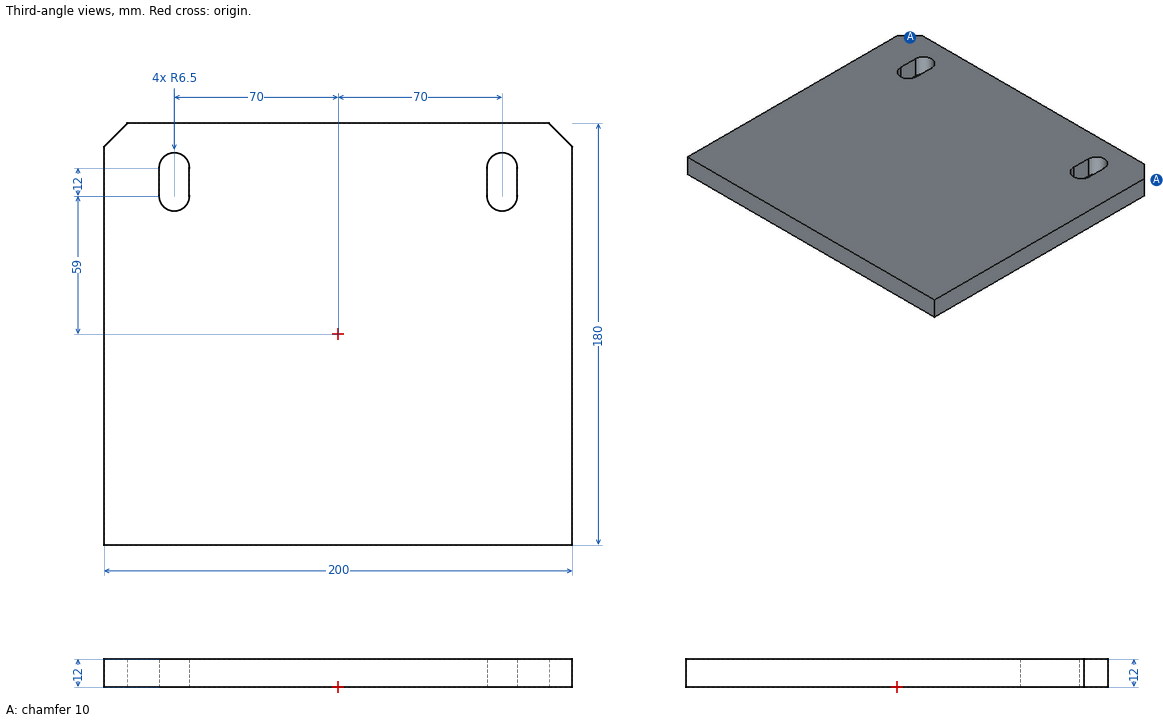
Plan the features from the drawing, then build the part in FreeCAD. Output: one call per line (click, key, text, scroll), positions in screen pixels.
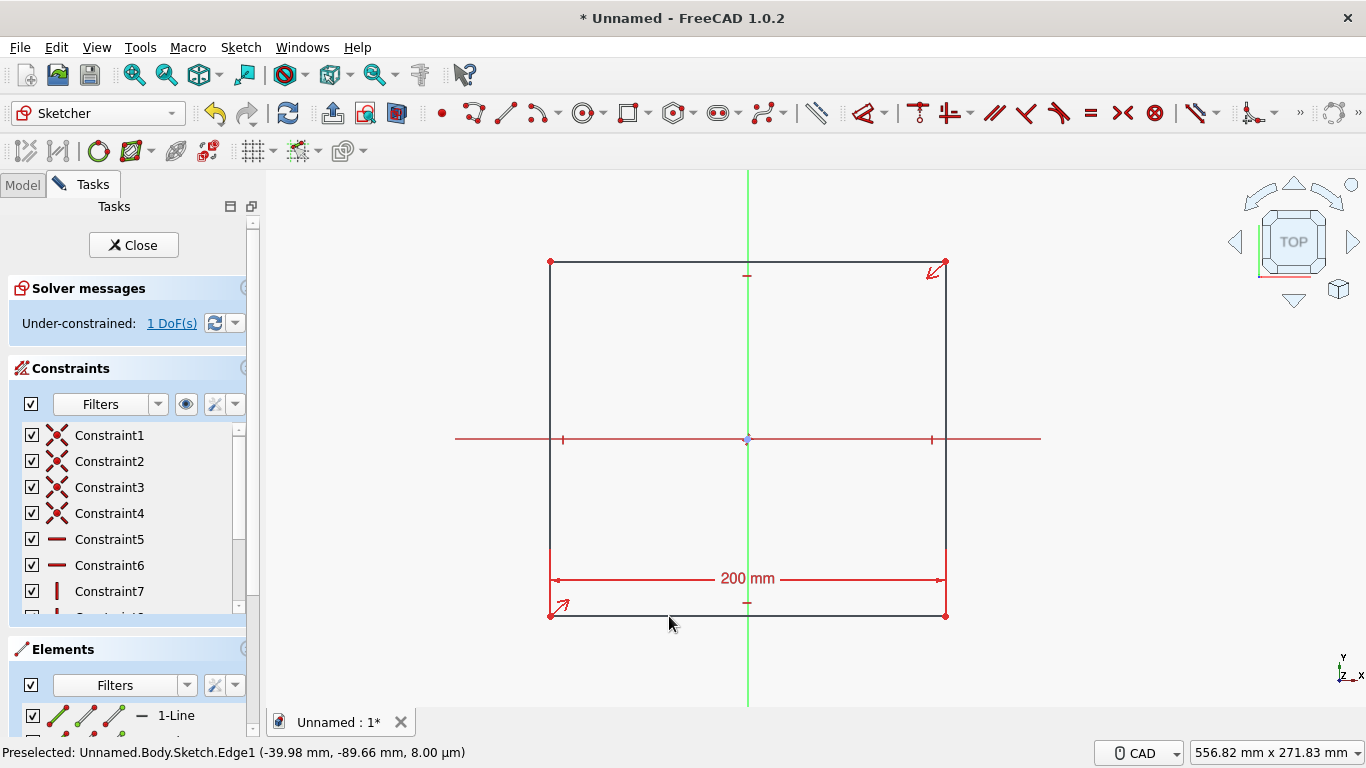
click(946, 510)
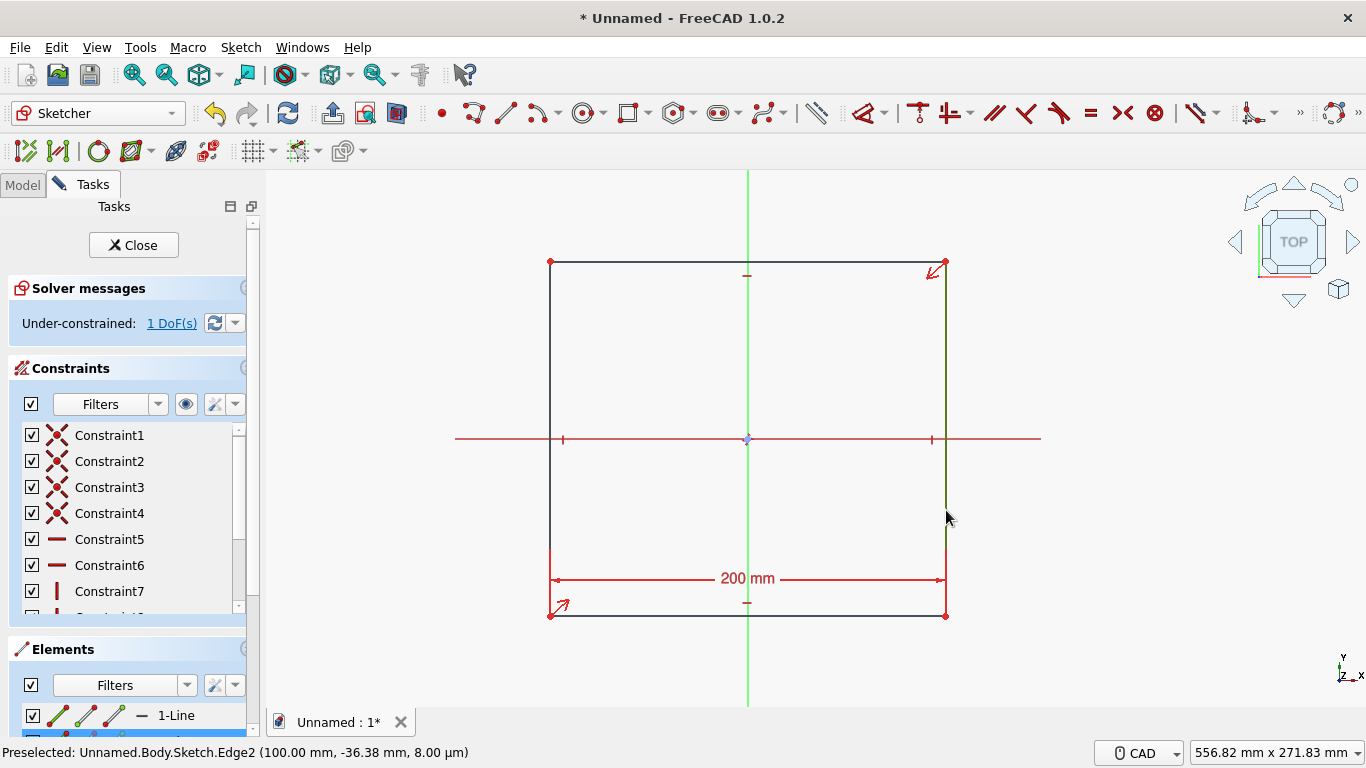
click(886, 114)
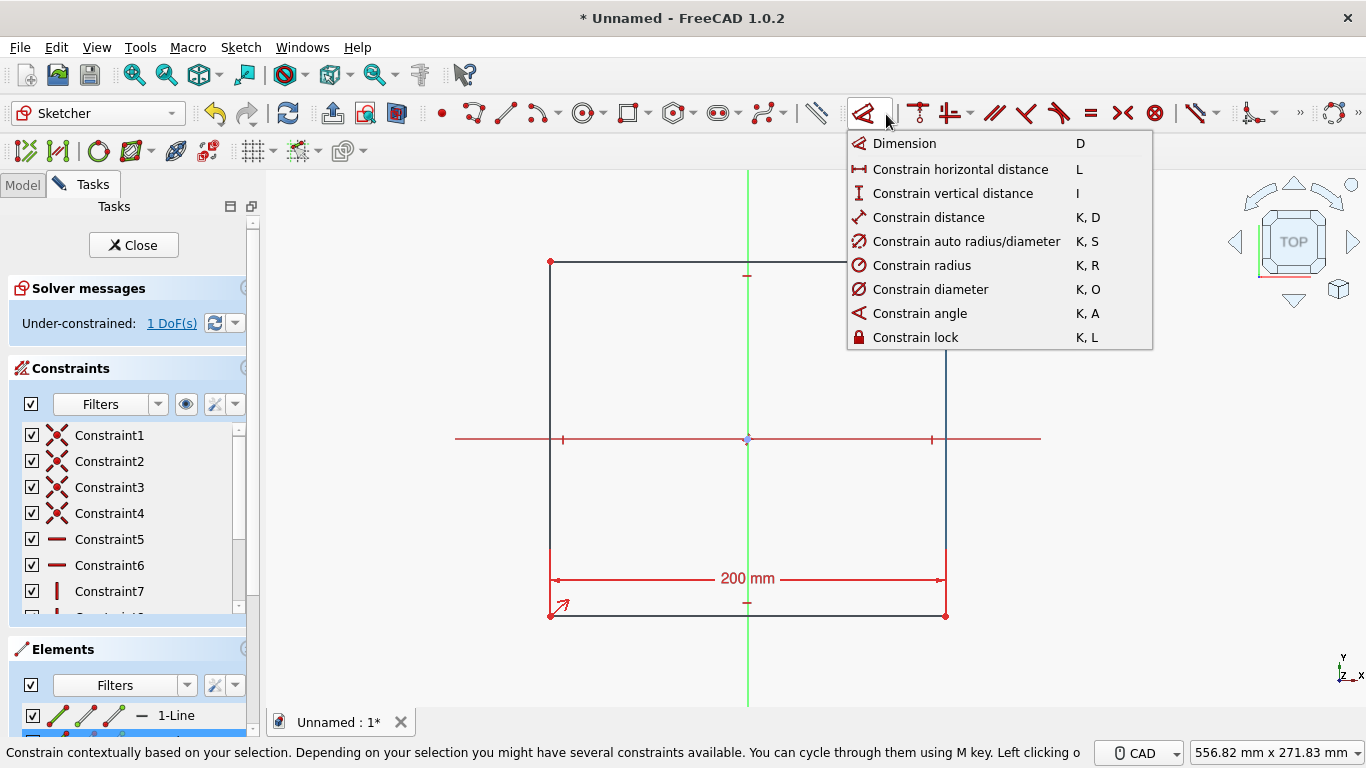
click(1000, 193)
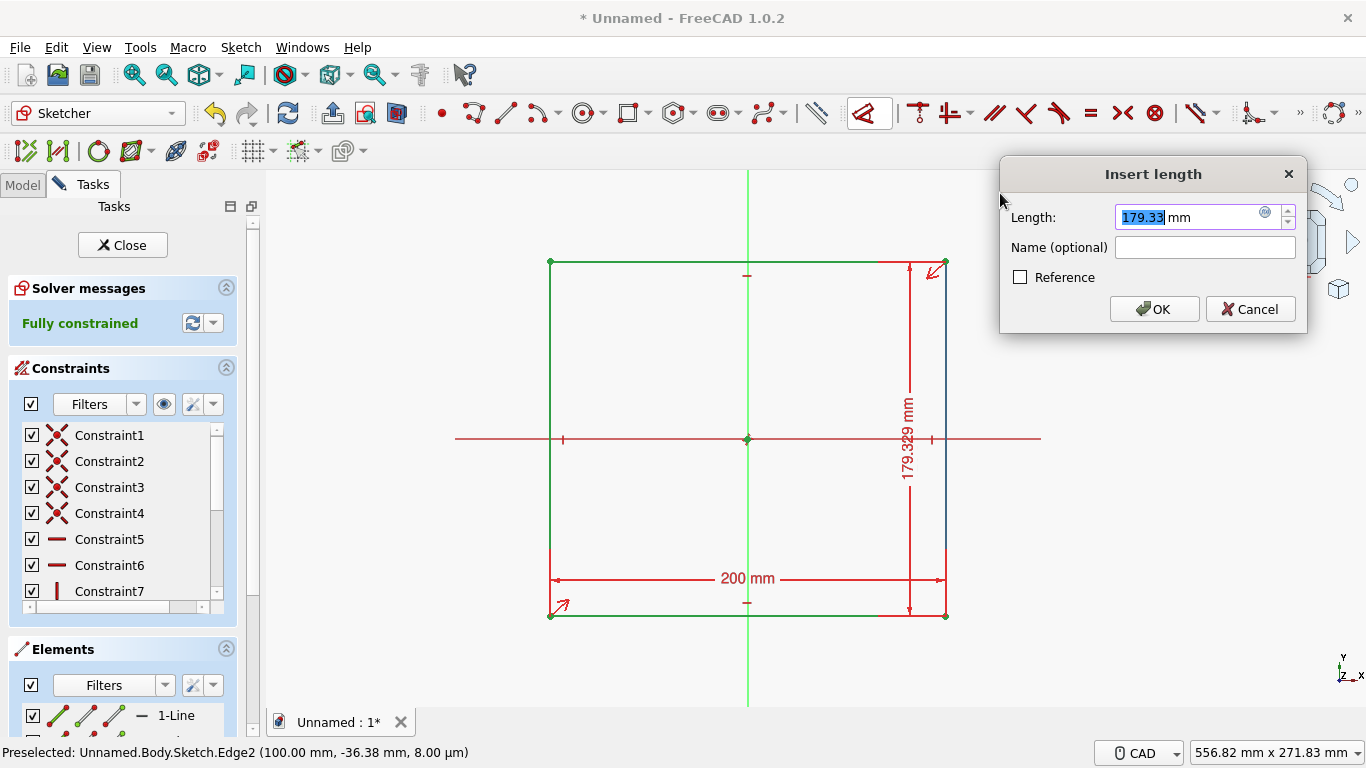
text(180)
key(Return)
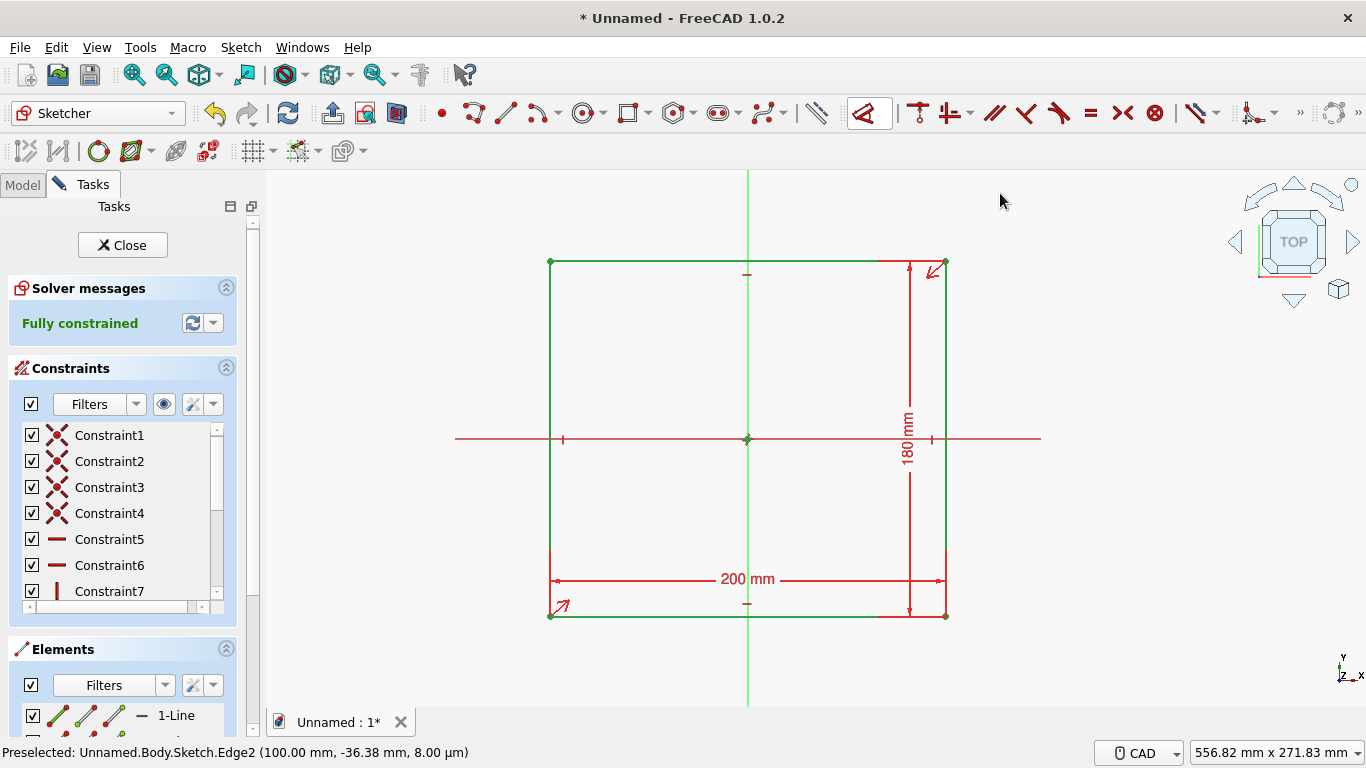
click(123, 245)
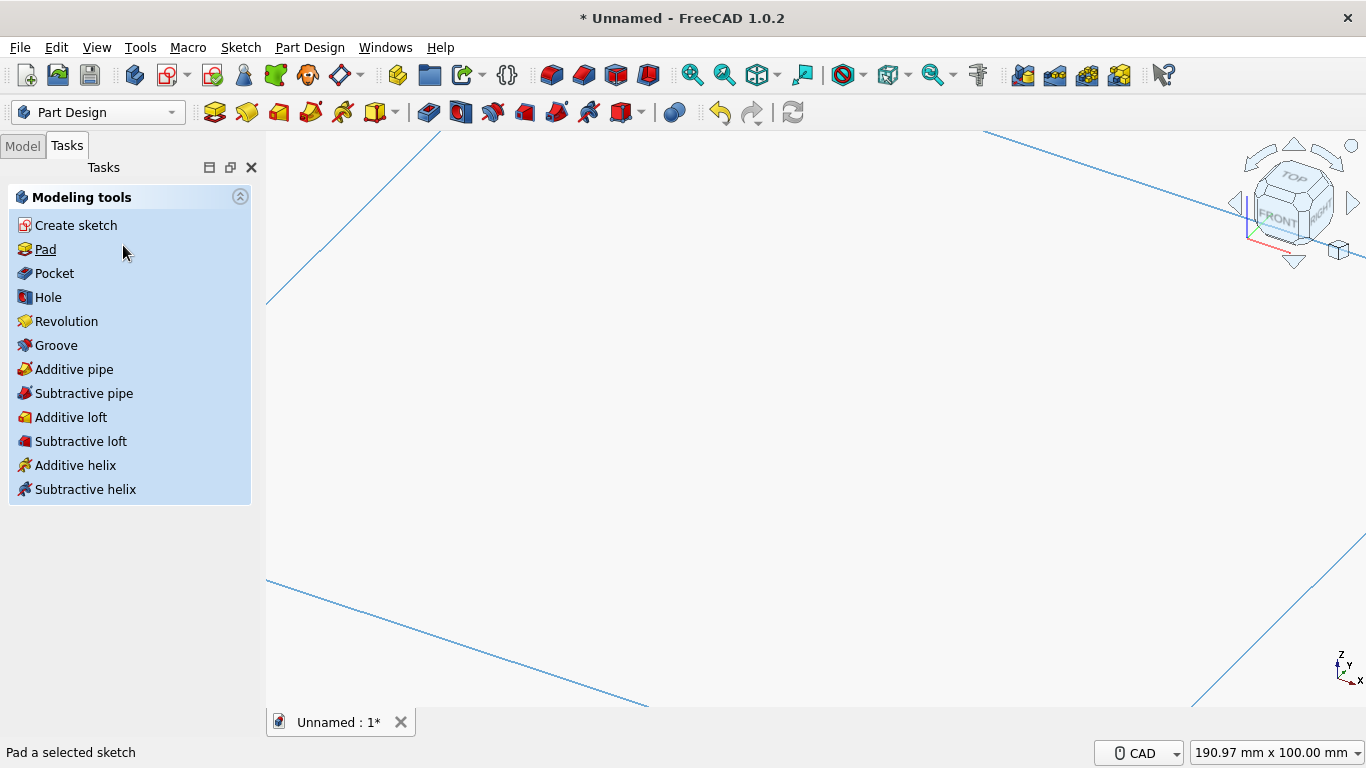
click(216, 112)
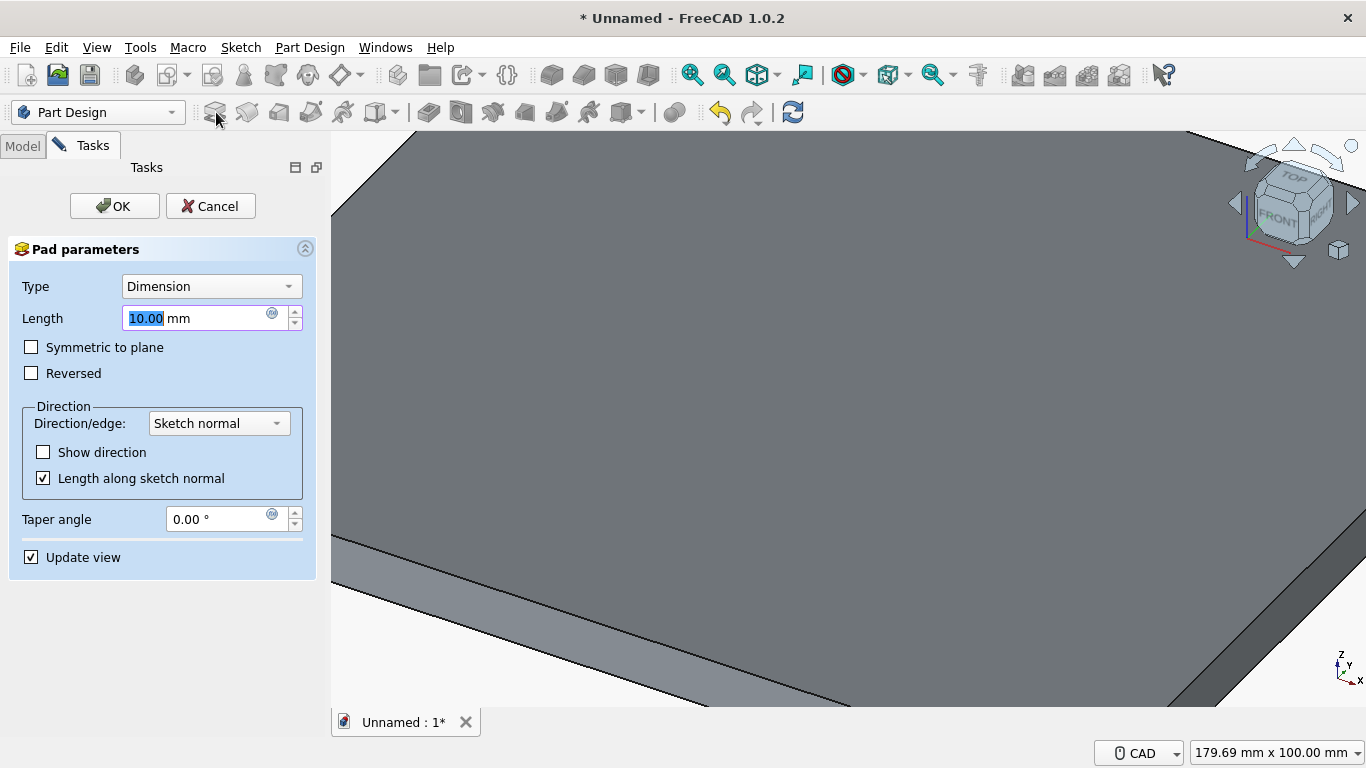
text(12)
key(Tab)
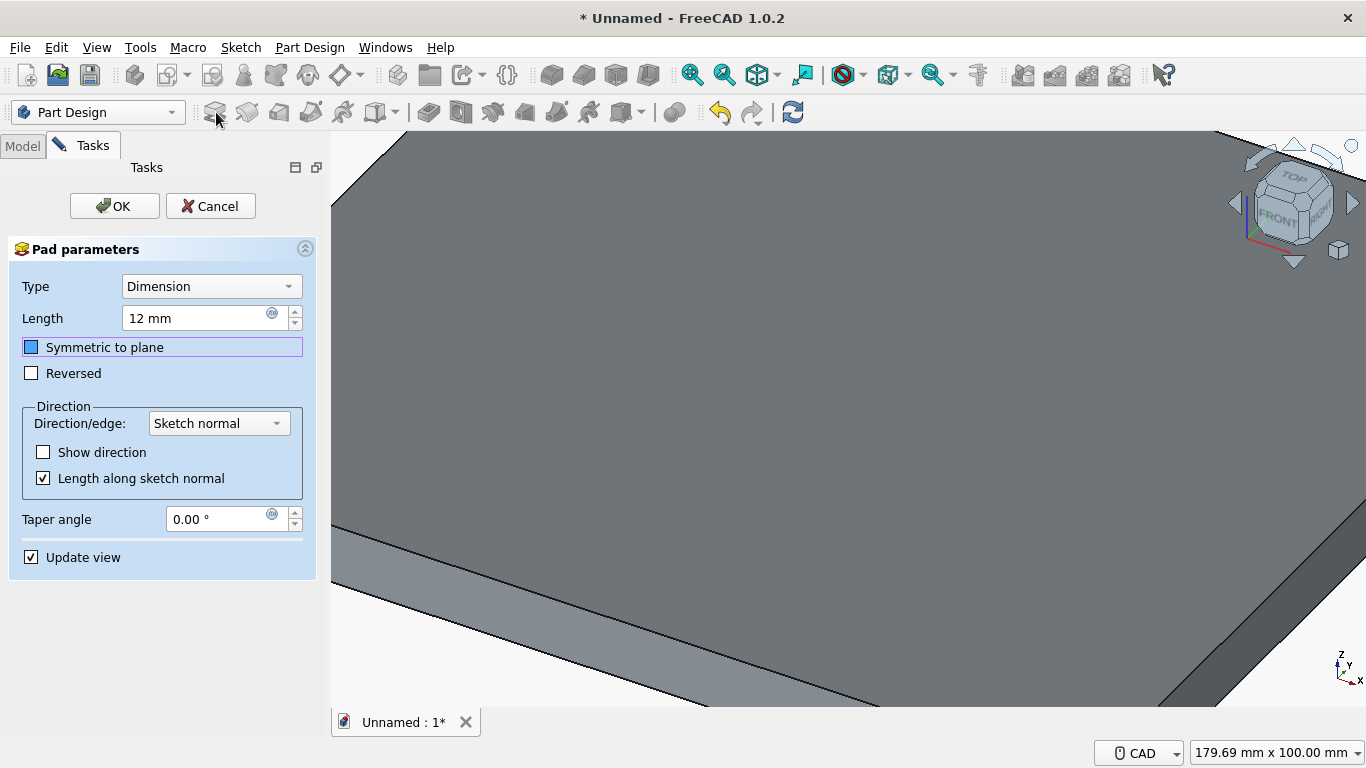
click(115, 206)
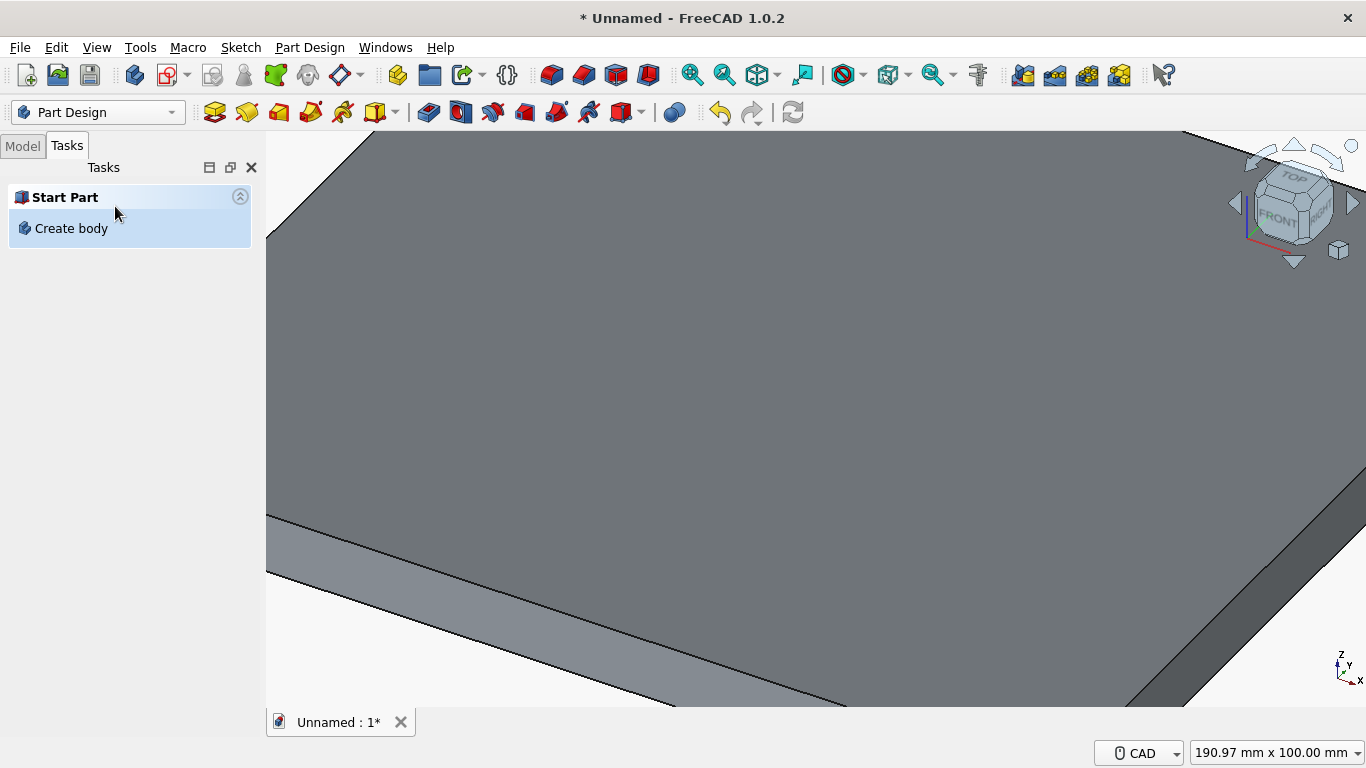
click(694, 76)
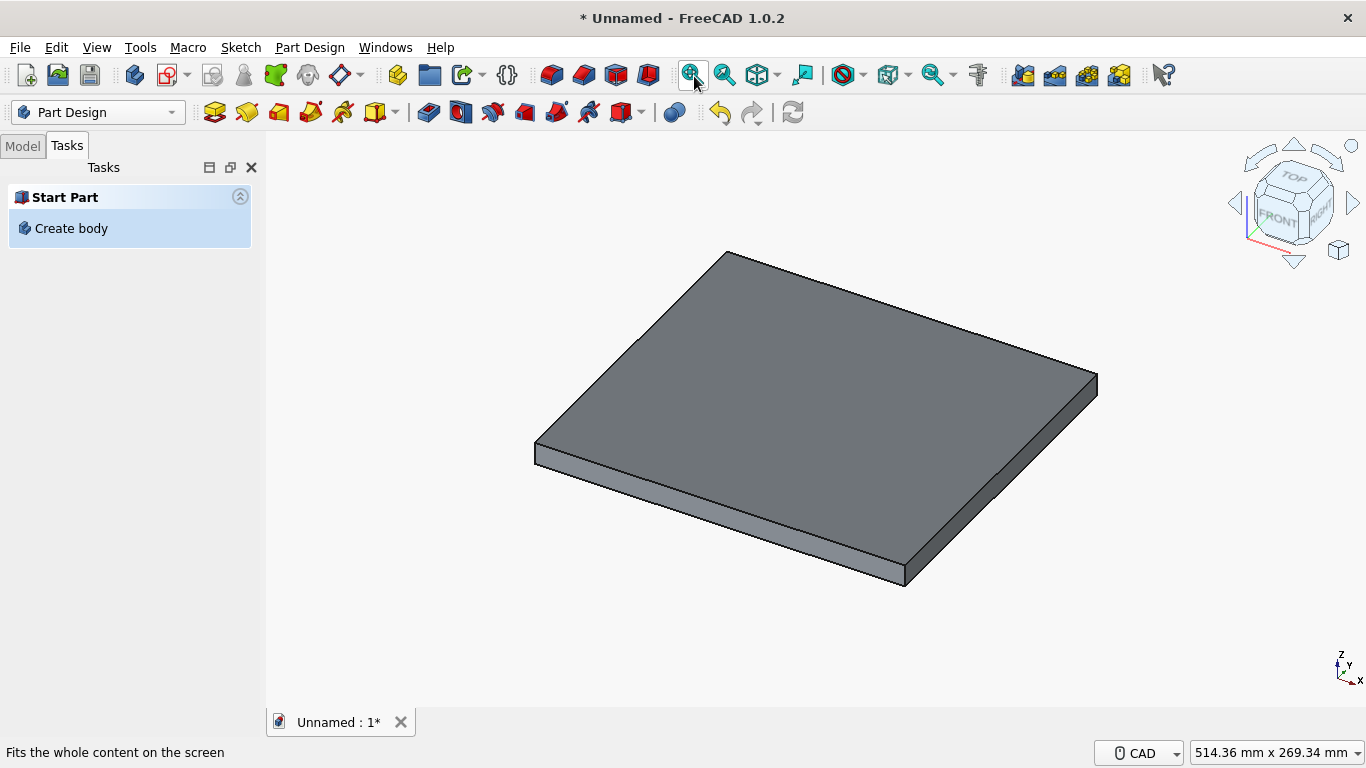
key(0)